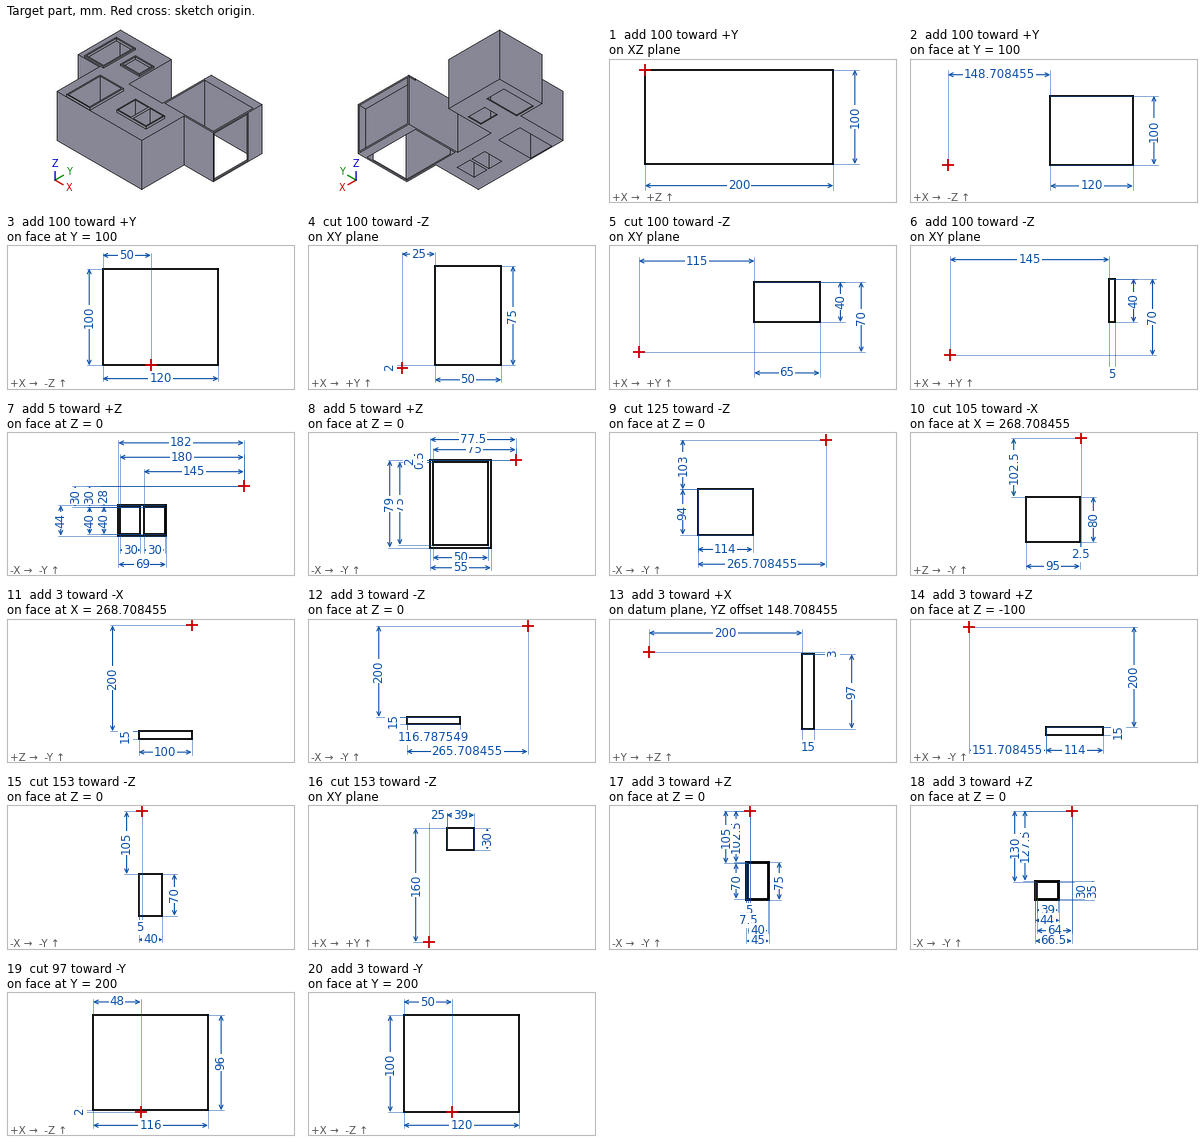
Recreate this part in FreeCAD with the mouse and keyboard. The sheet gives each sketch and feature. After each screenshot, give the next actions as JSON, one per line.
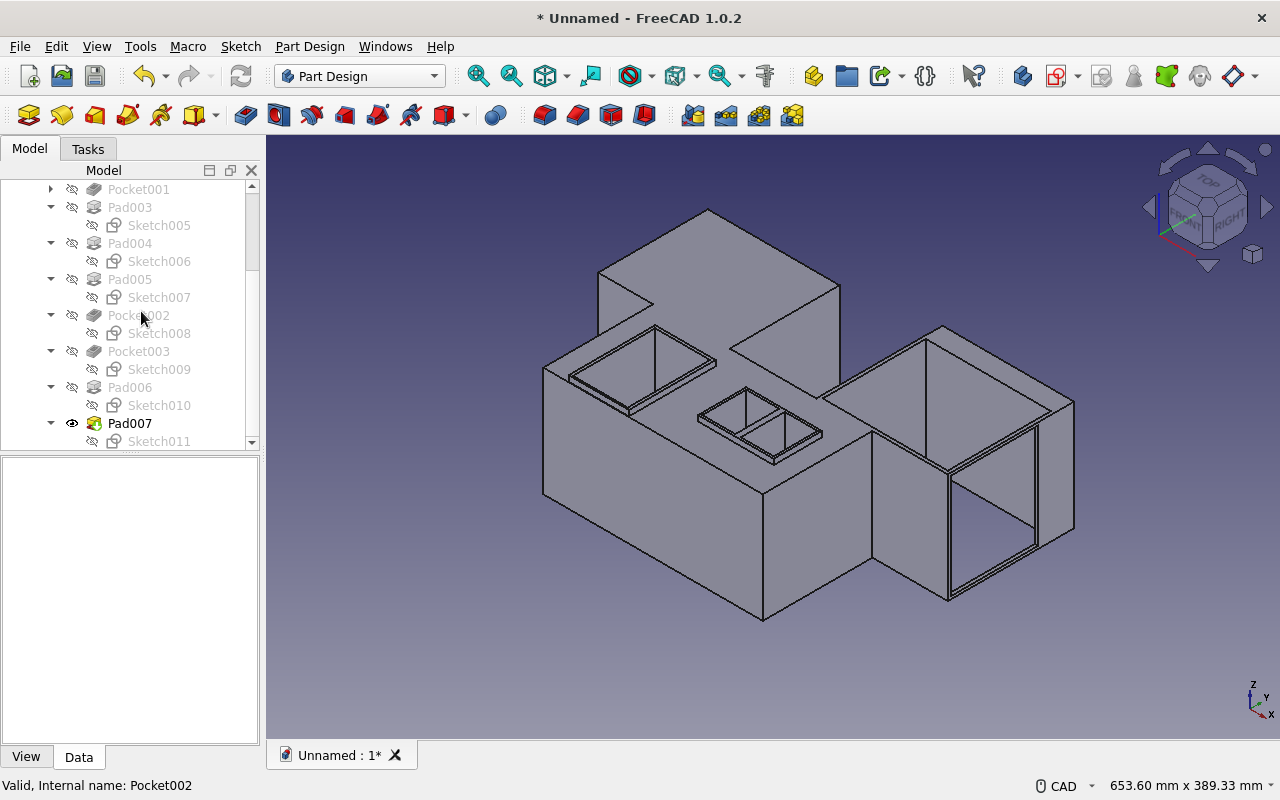
{"action": "scroll", "coordinate": [141, 311], "scroll_direction": "up", "scroll_amount": 15}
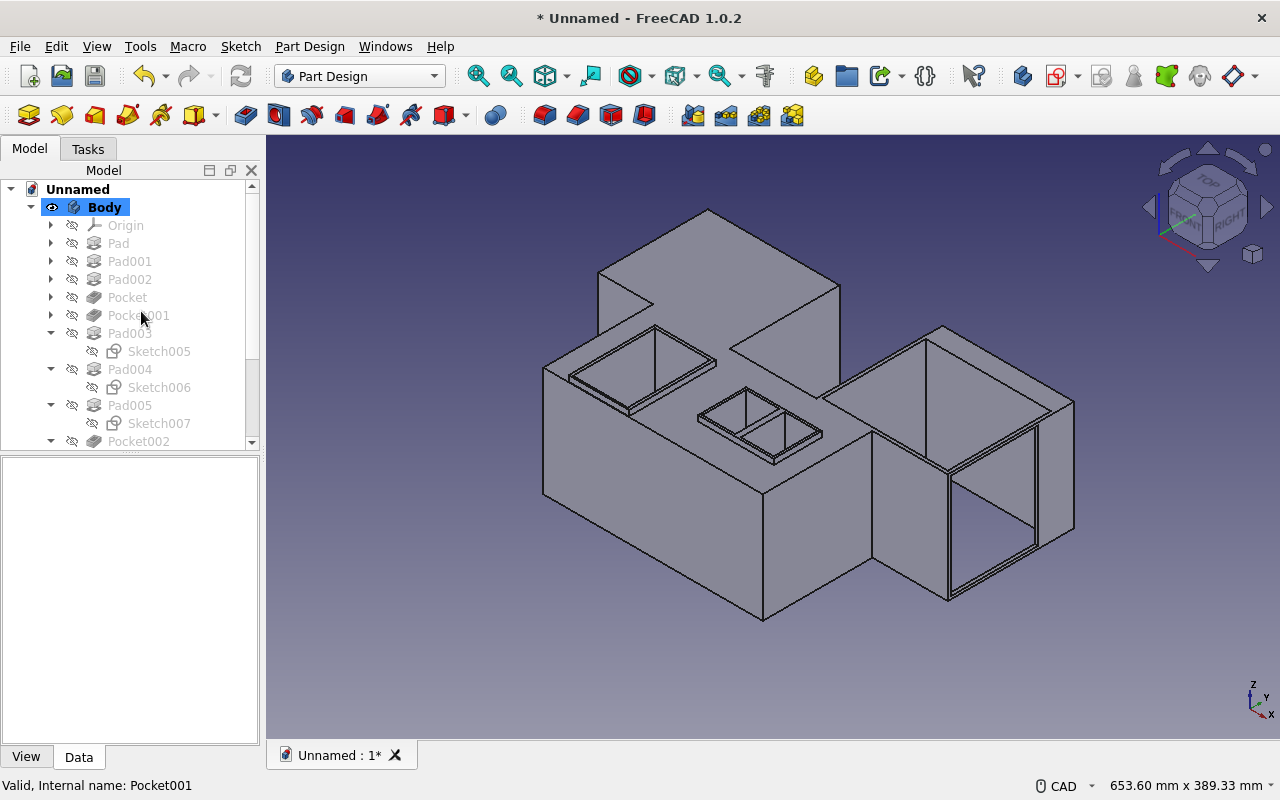
{"action": "left_click", "coordinate": [51, 225]}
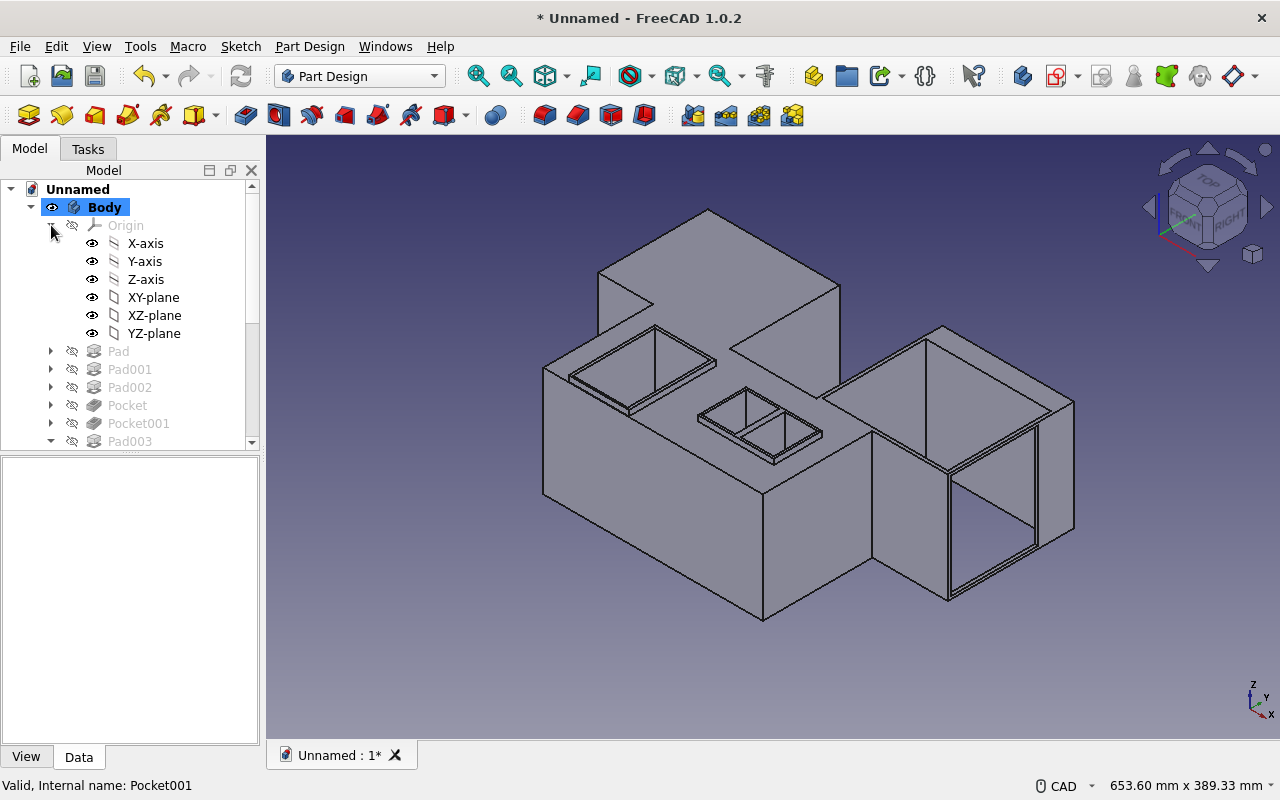
{"action": "left_click", "coordinate": [137, 333]}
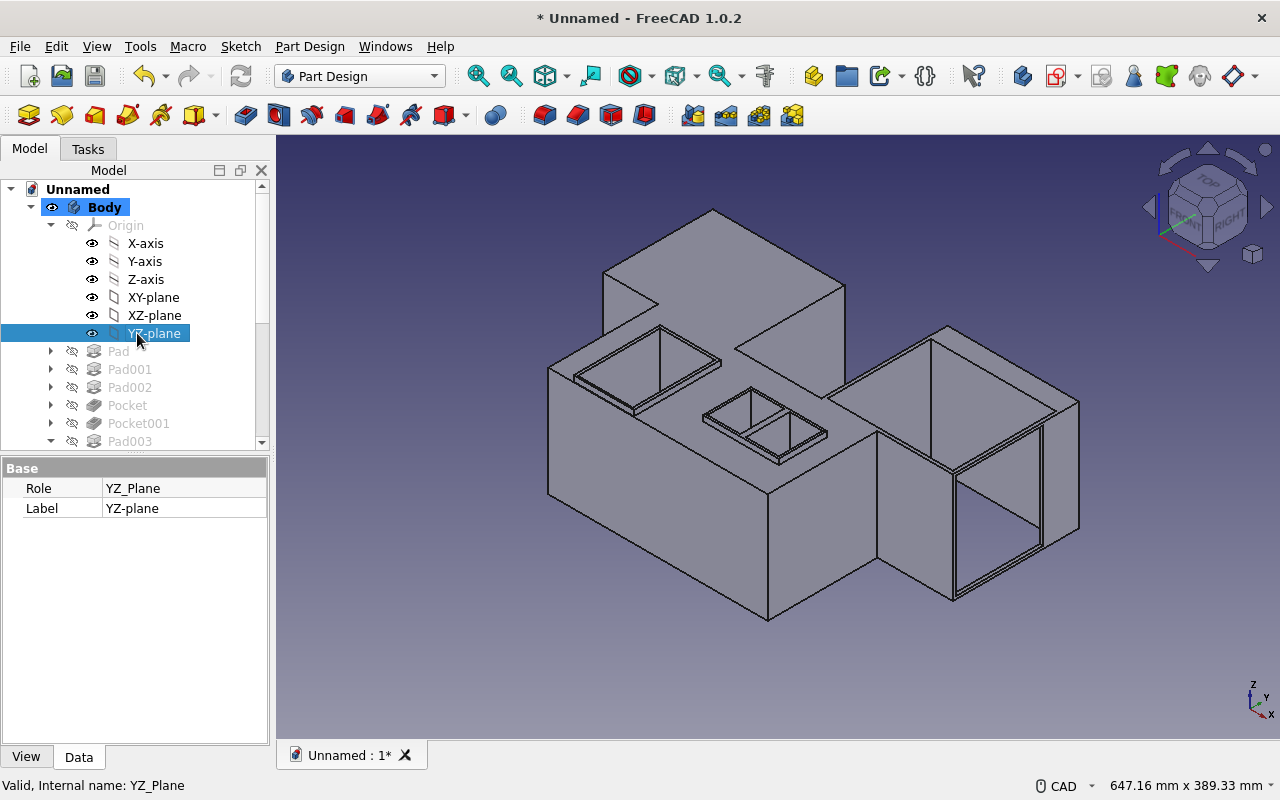
{"action": "left_click", "coordinate": [1232, 76]}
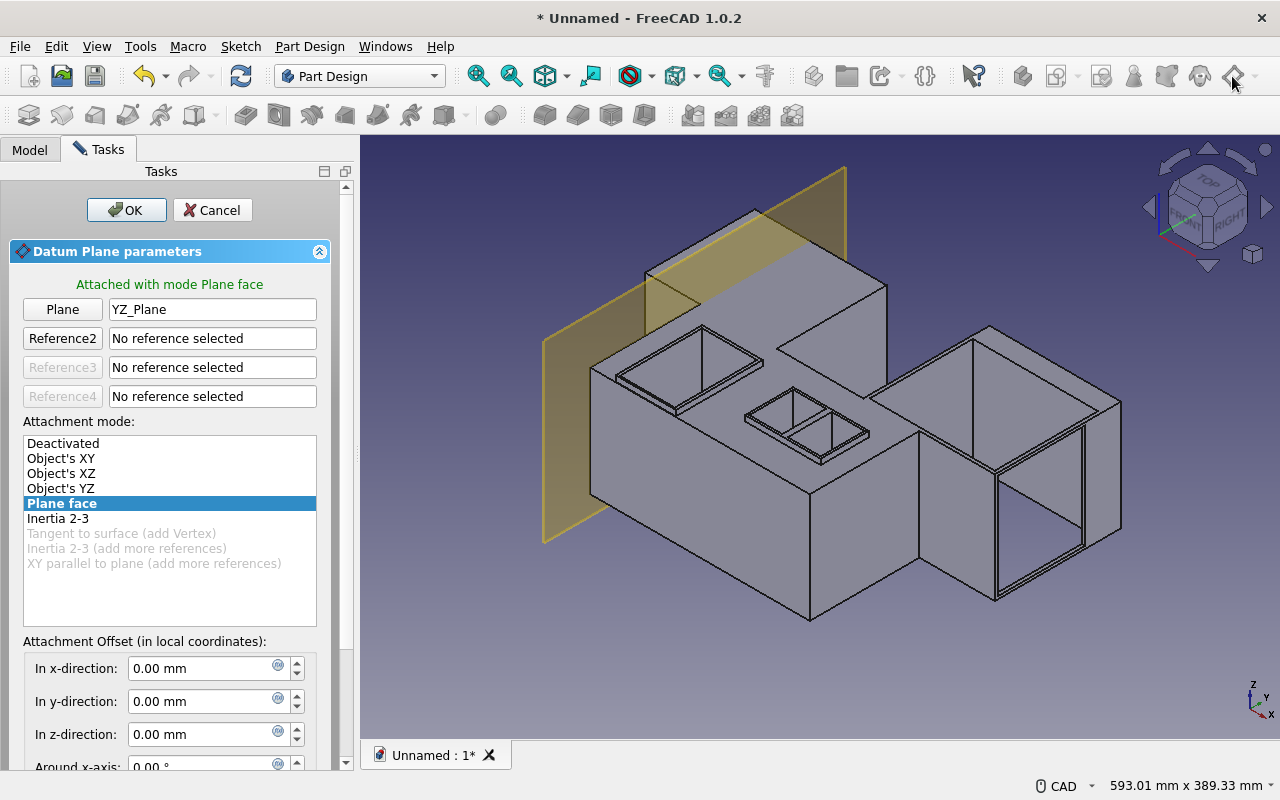
{"action": "triple_click", "coordinate": [210, 734]}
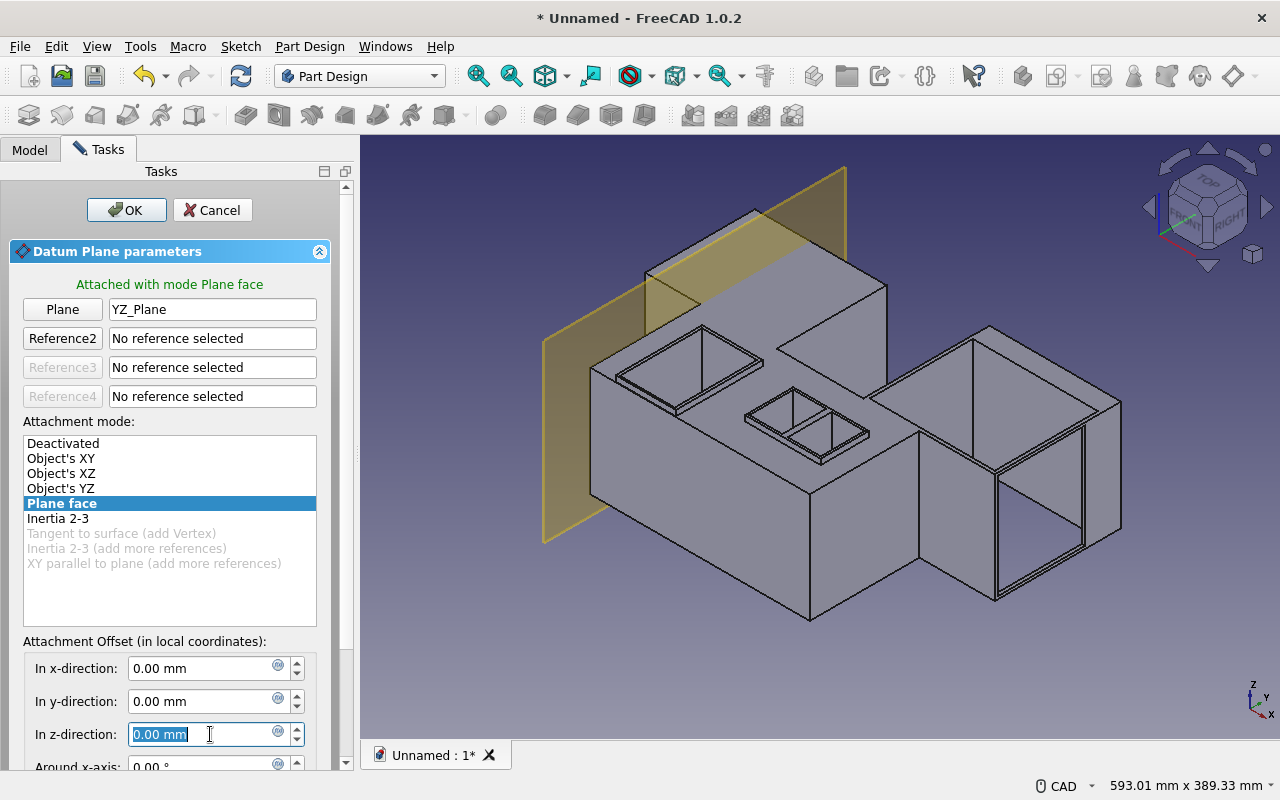
{"action": "type", "text": "148.708455"}
{"action": "key", "text": "Tab"}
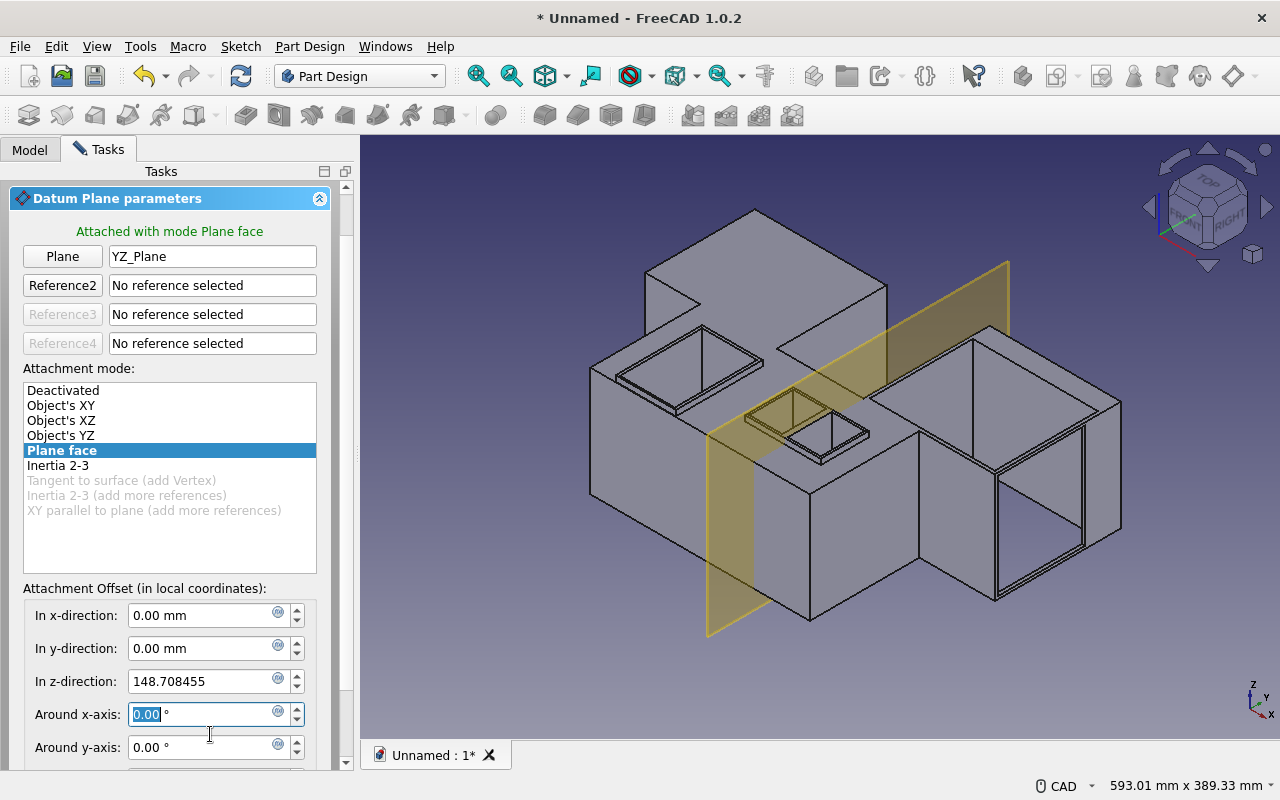
{"action": "scroll", "coordinate": [346, 476], "scroll_direction": "up", "scroll_amount": 2}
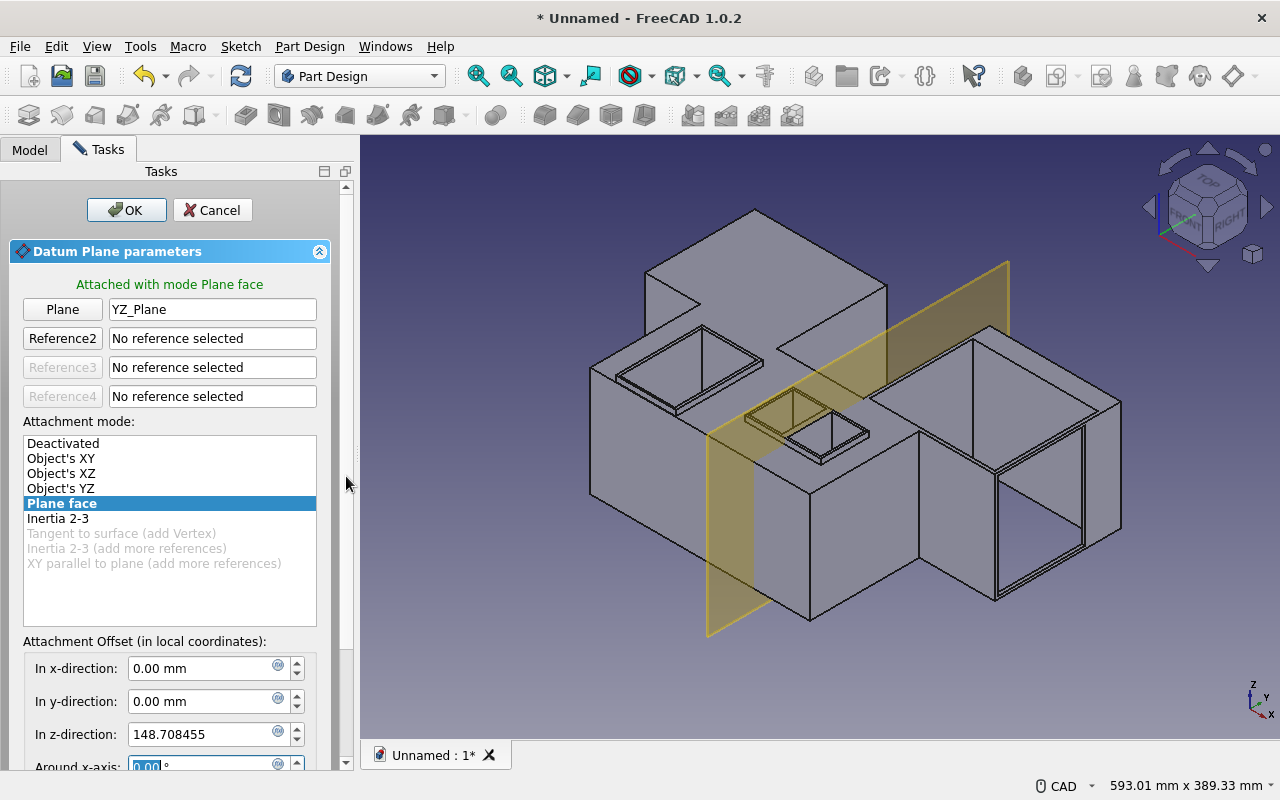
{"action": "left_click", "coordinate": [127, 210]}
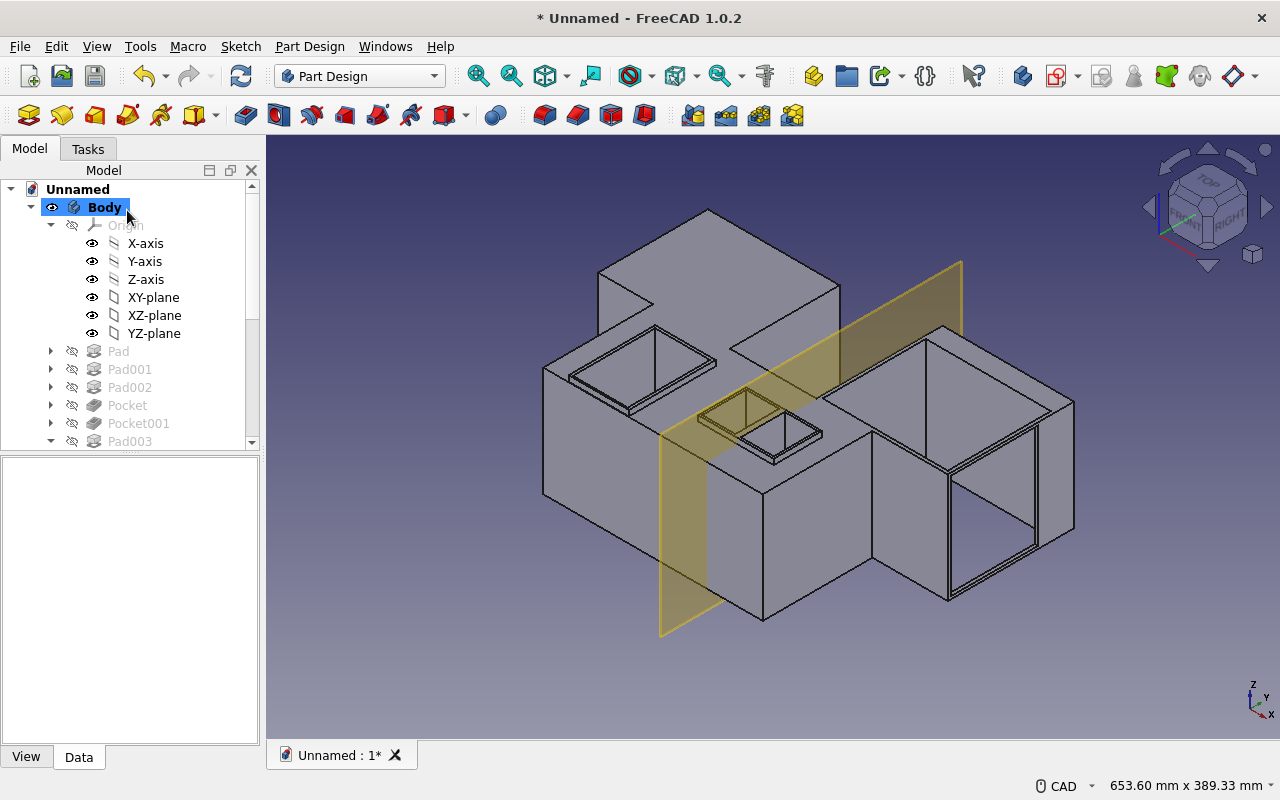
{"action": "scroll", "coordinate": [101, 311], "scroll_direction": "down", "scroll_amount": 3}